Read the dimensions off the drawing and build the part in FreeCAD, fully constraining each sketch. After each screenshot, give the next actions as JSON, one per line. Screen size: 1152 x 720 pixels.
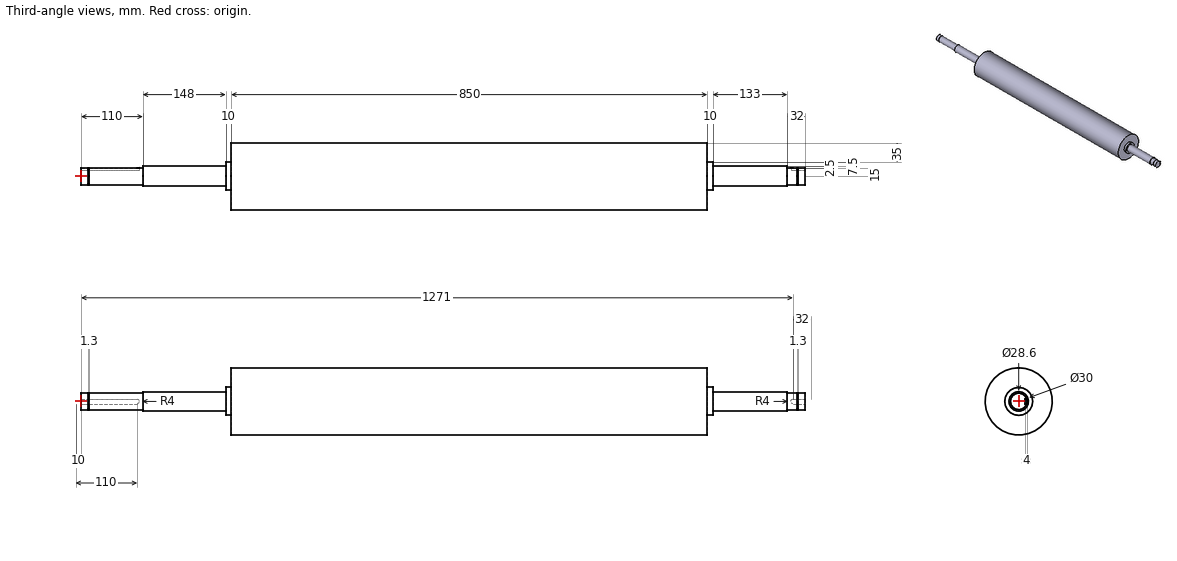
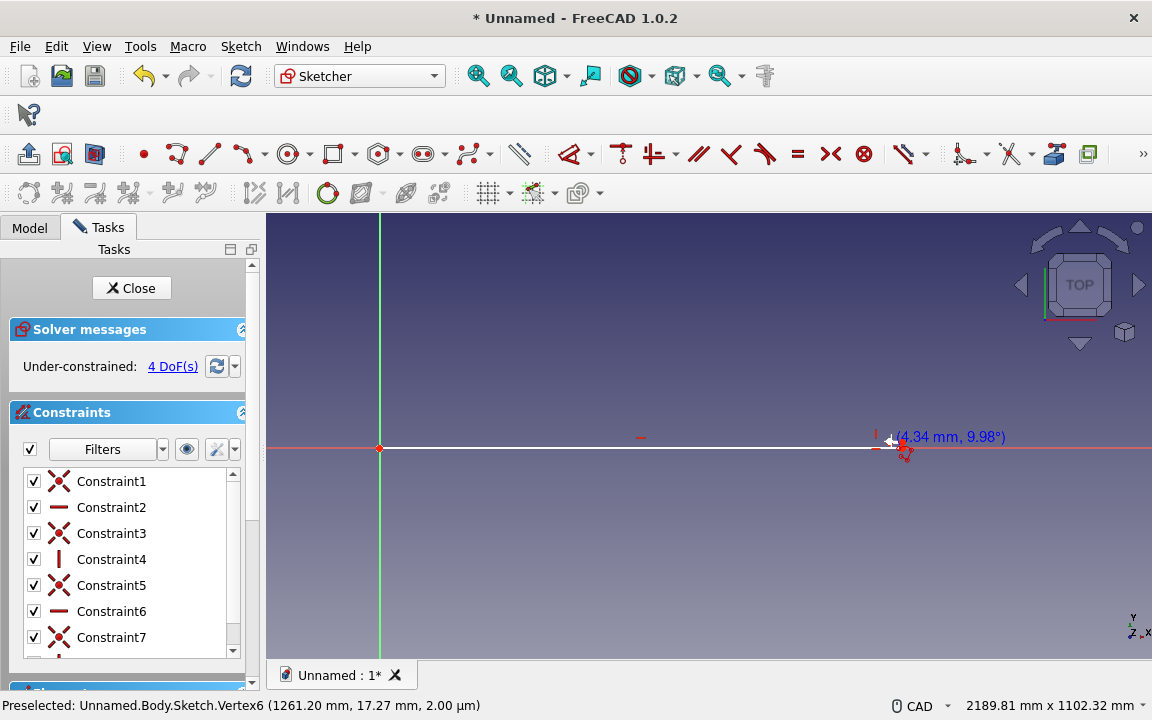
{"action": "scroll", "coordinate": [836, 441], "scroll_direction": "up", "scroll_amount": 5}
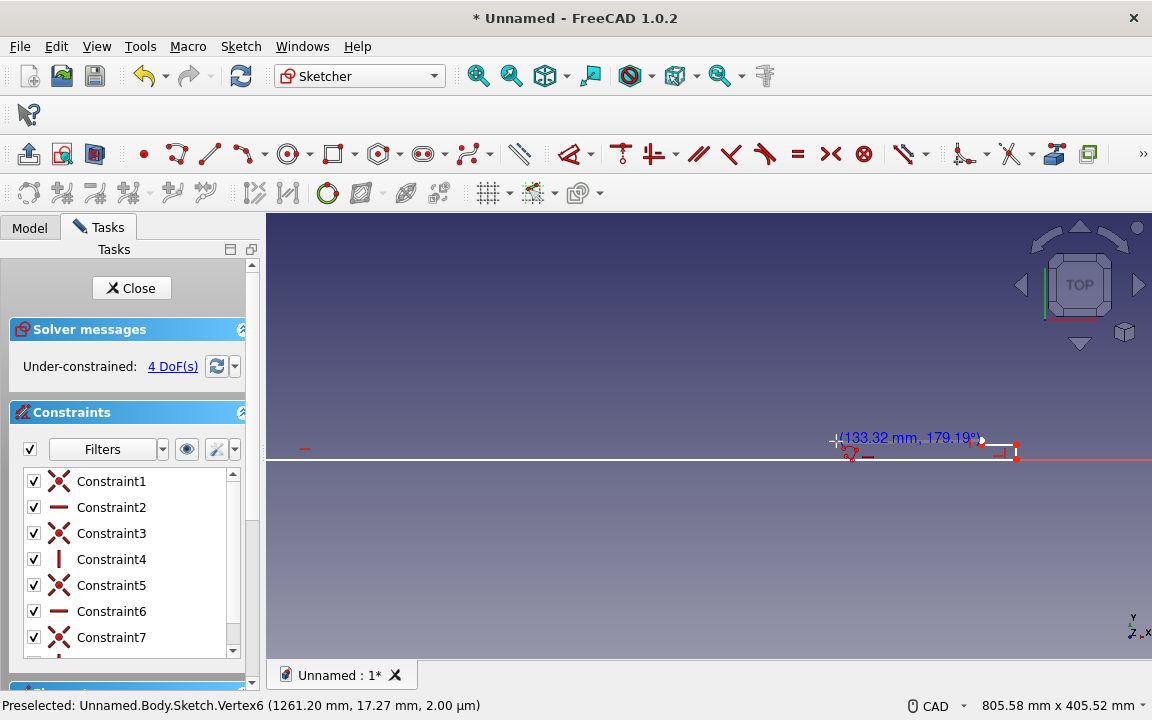
{"action": "left_click", "coordinate": [835, 441]}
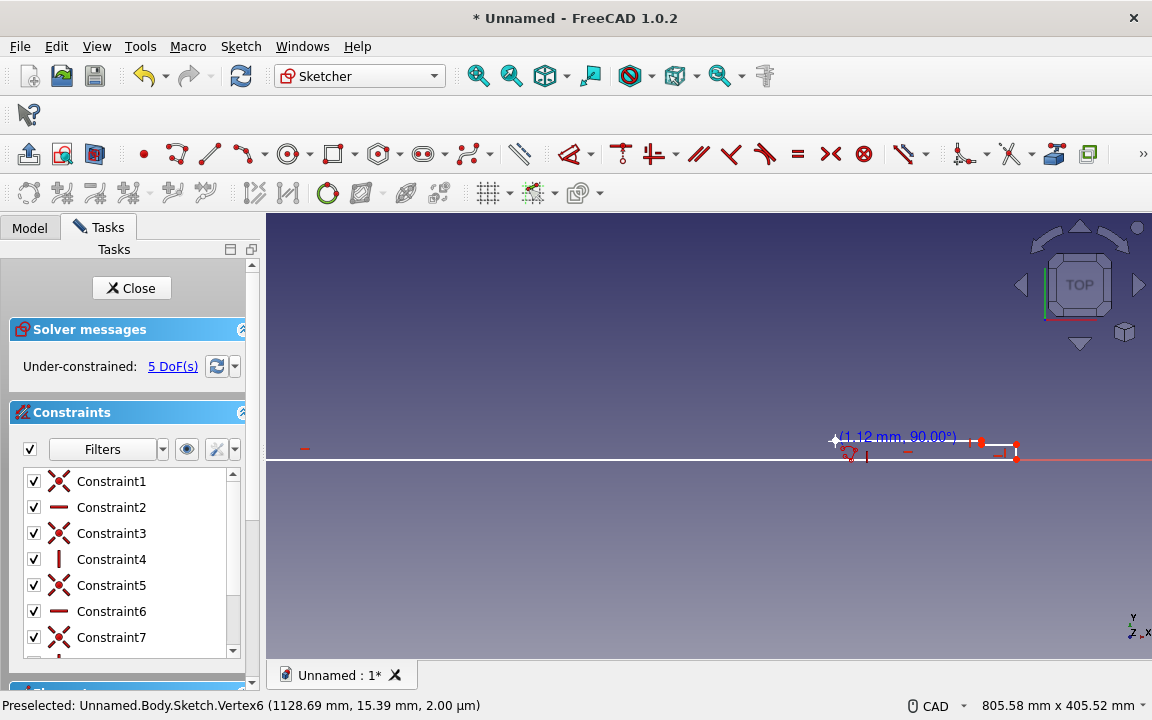
{"action": "scroll", "coordinate": [835, 432], "scroll_direction": "up", "scroll_amount": 4}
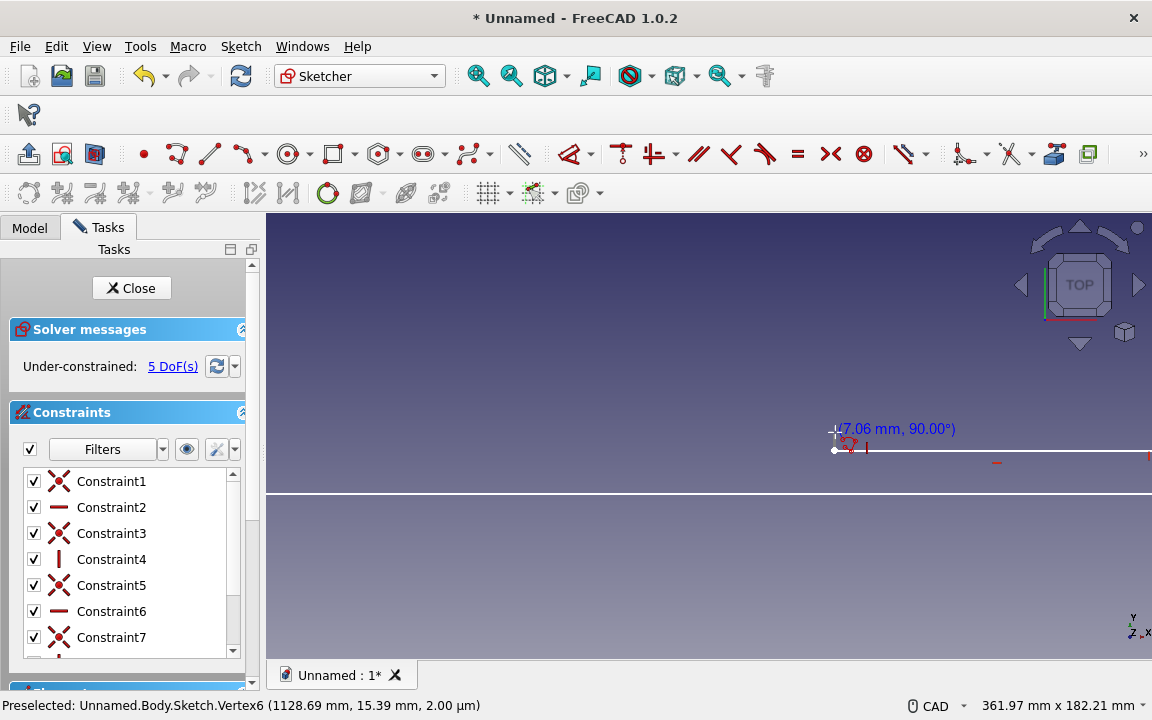
{"action": "left_click", "coordinate": [834, 432]}
{"action": "left_click", "coordinate": [810, 432]}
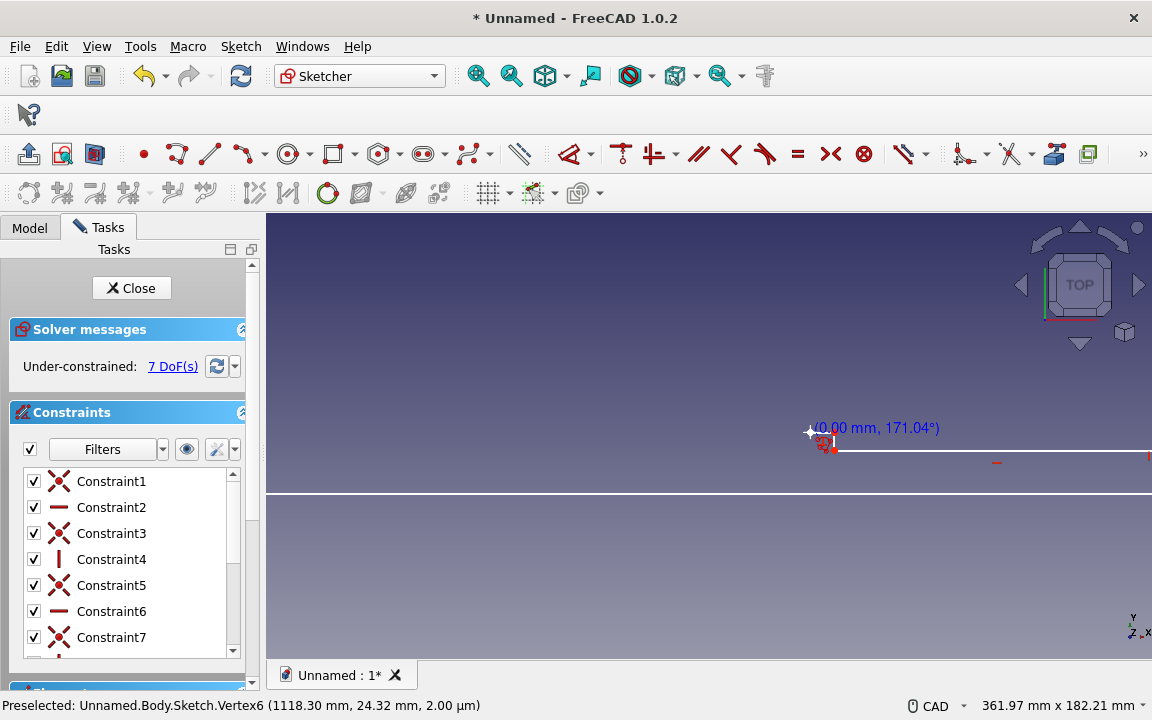
{"action": "scroll", "coordinate": [835, 439], "scroll_direction": "down", "scroll_amount": 9}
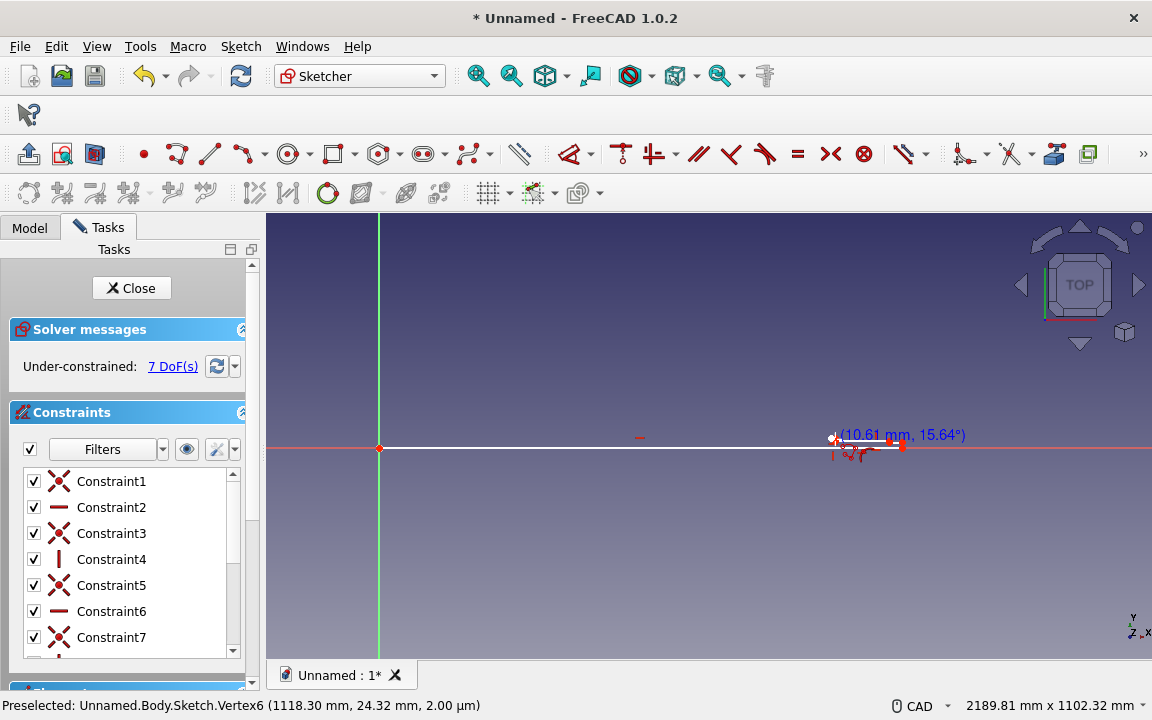
{"action": "left_click", "coordinate": [831, 424]}
{"action": "left_click", "coordinate": [488, 424]}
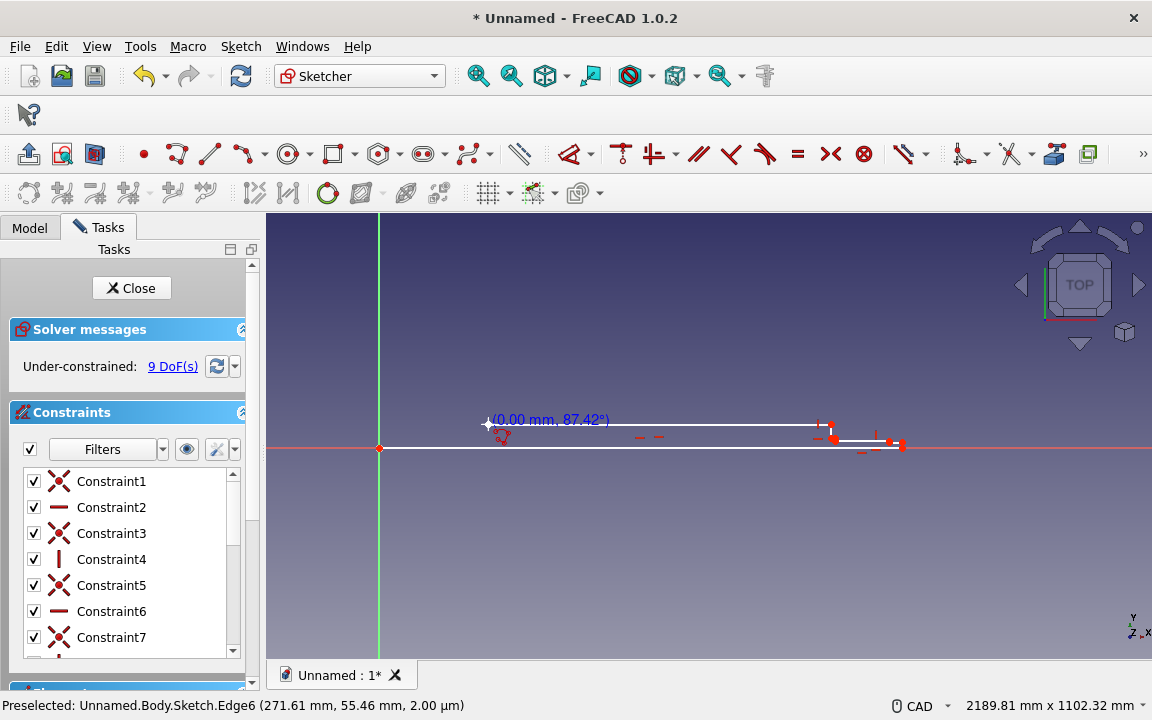
{"action": "scroll", "coordinate": [488, 438], "scroll_direction": "up", "scroll_amount": 3}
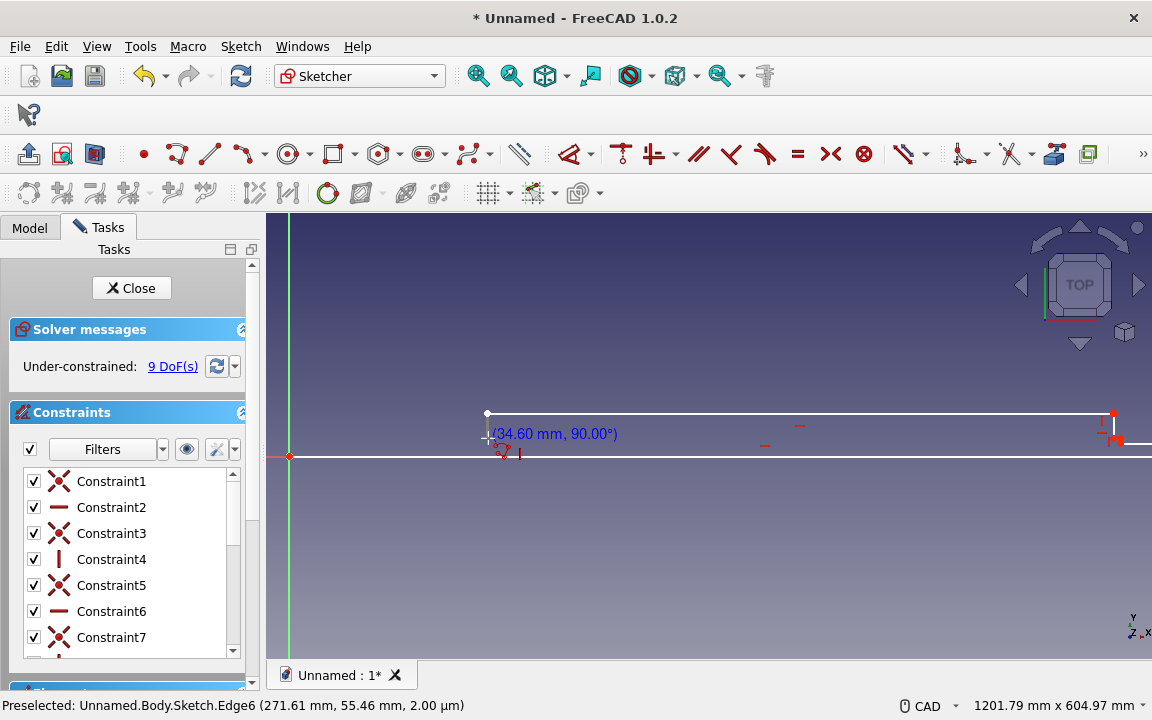
{"action": "left_click", "coordinate": [488, 438]}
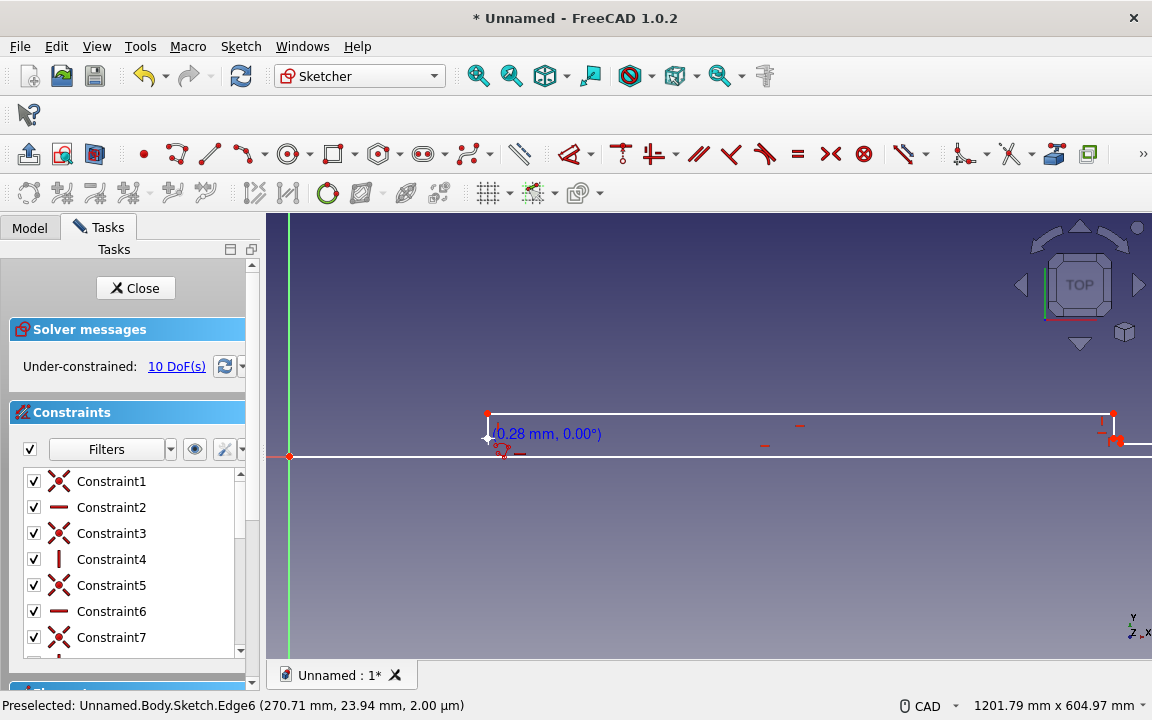
{"action": "scroll", "coordinate": [480, 438], "scroll_direction": "up", "scroll_amount": 4}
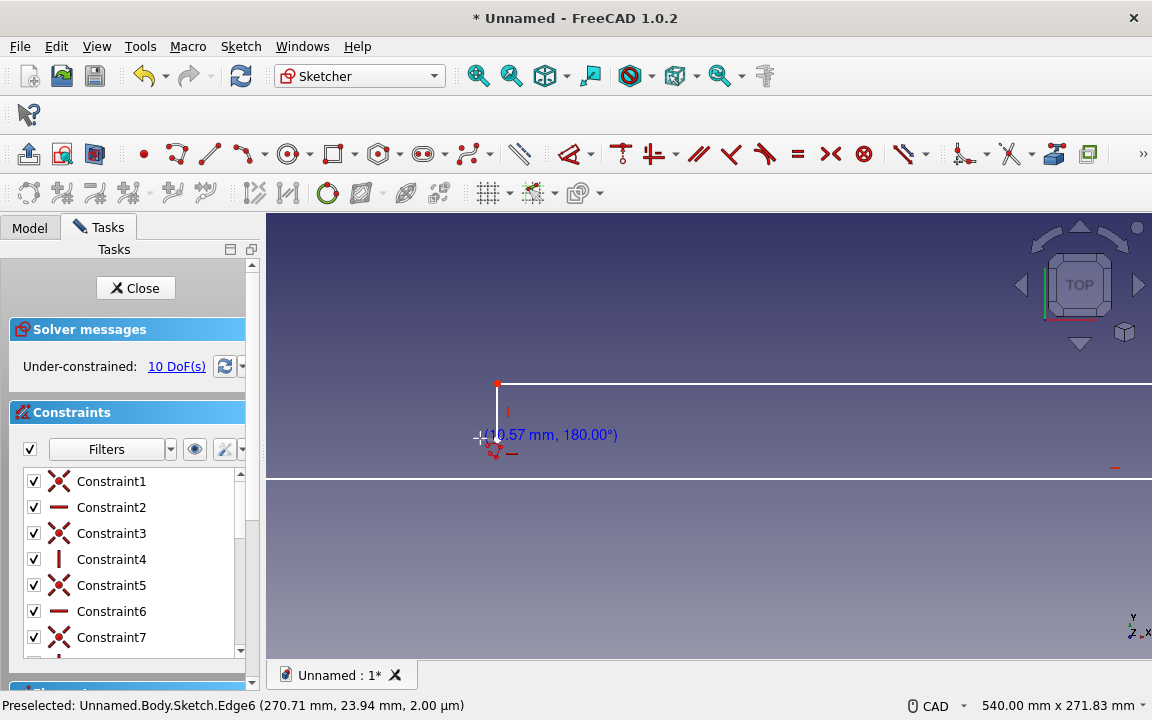
{"action": "left_click", "coordinate": [479, 437]}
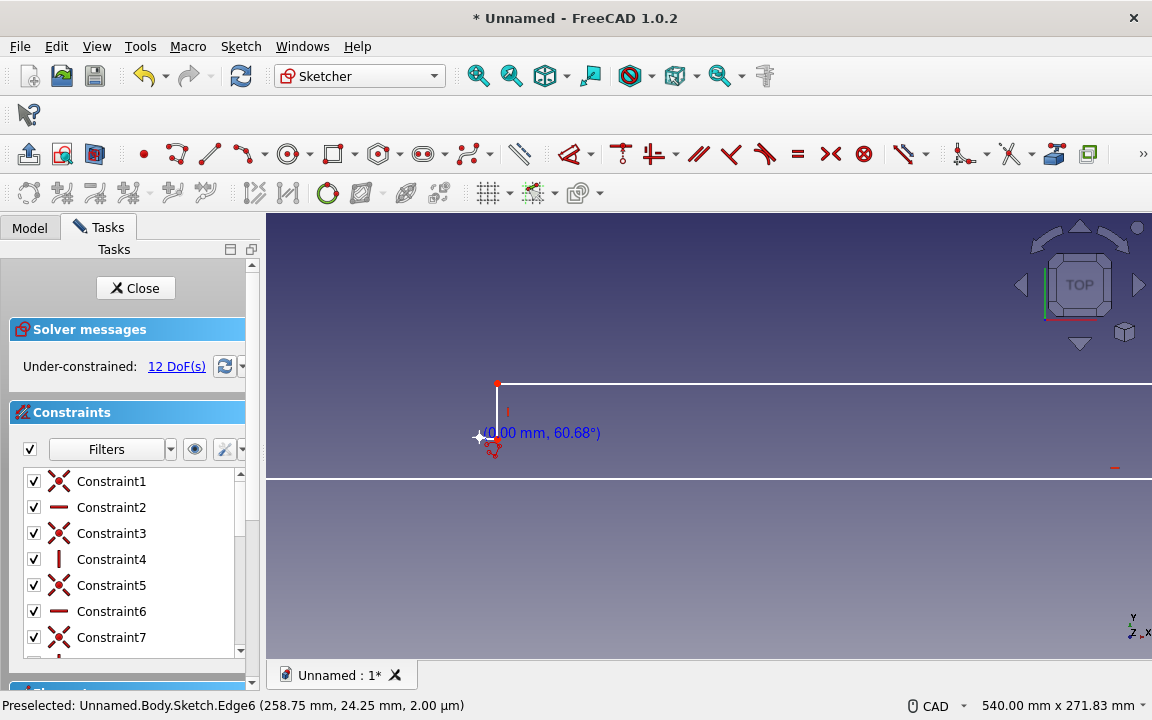
{"action": "scroll", "coordinate": [479, 450], "scroll_direction": "up", "scroll_amount": 2}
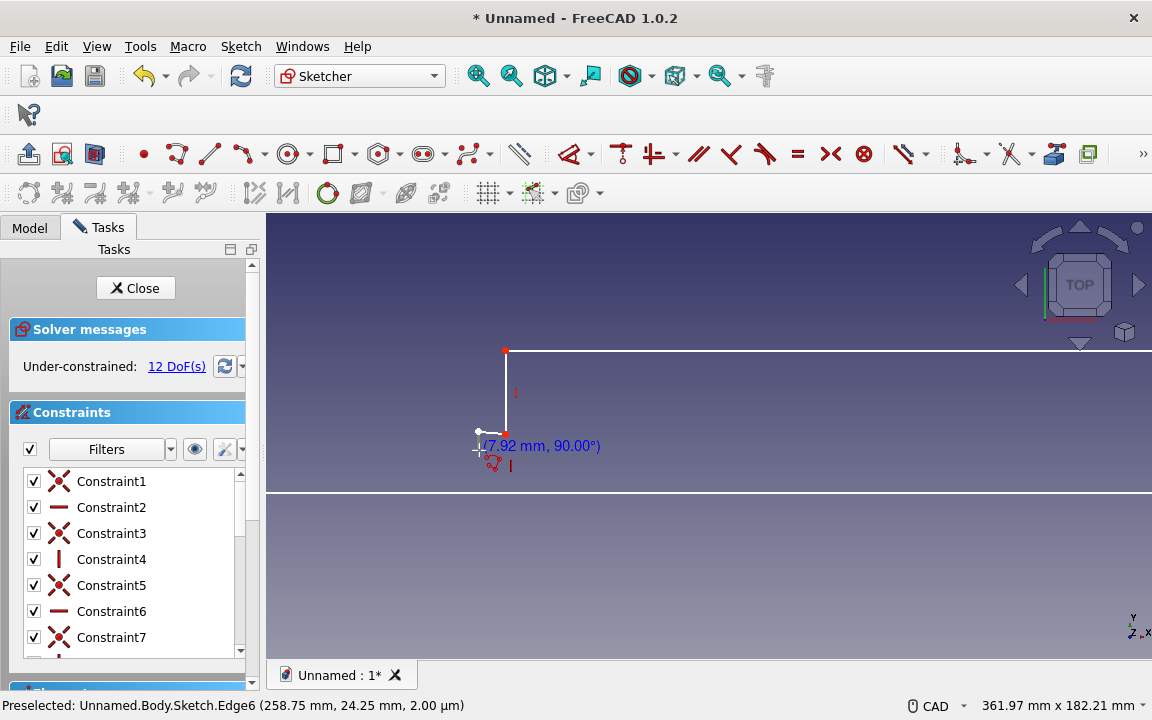
{"action": "left_click", "coordinate": [479, 450]}